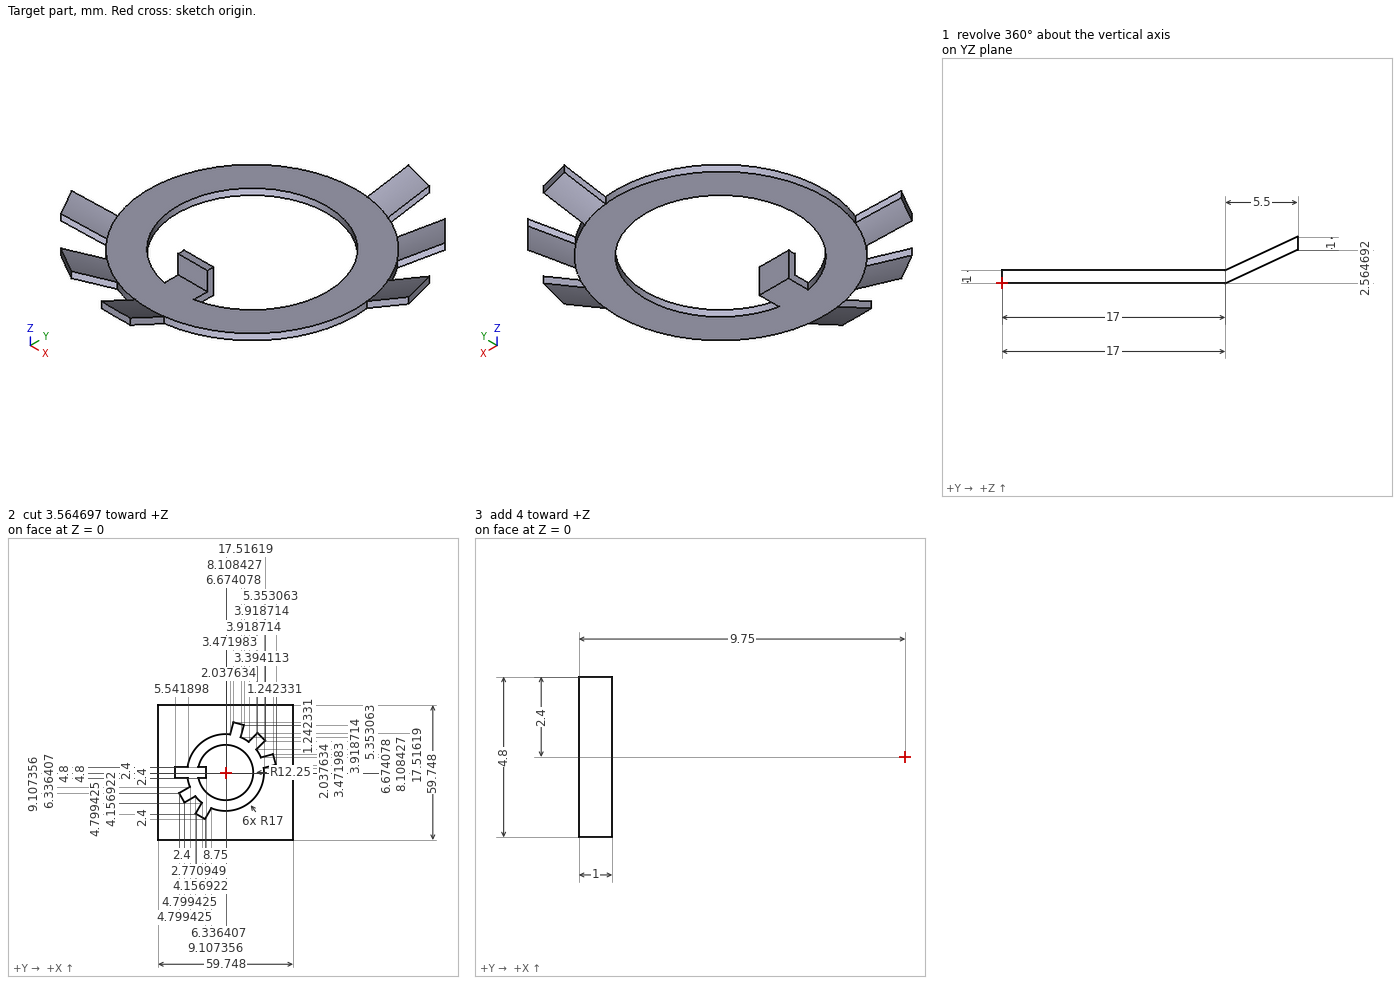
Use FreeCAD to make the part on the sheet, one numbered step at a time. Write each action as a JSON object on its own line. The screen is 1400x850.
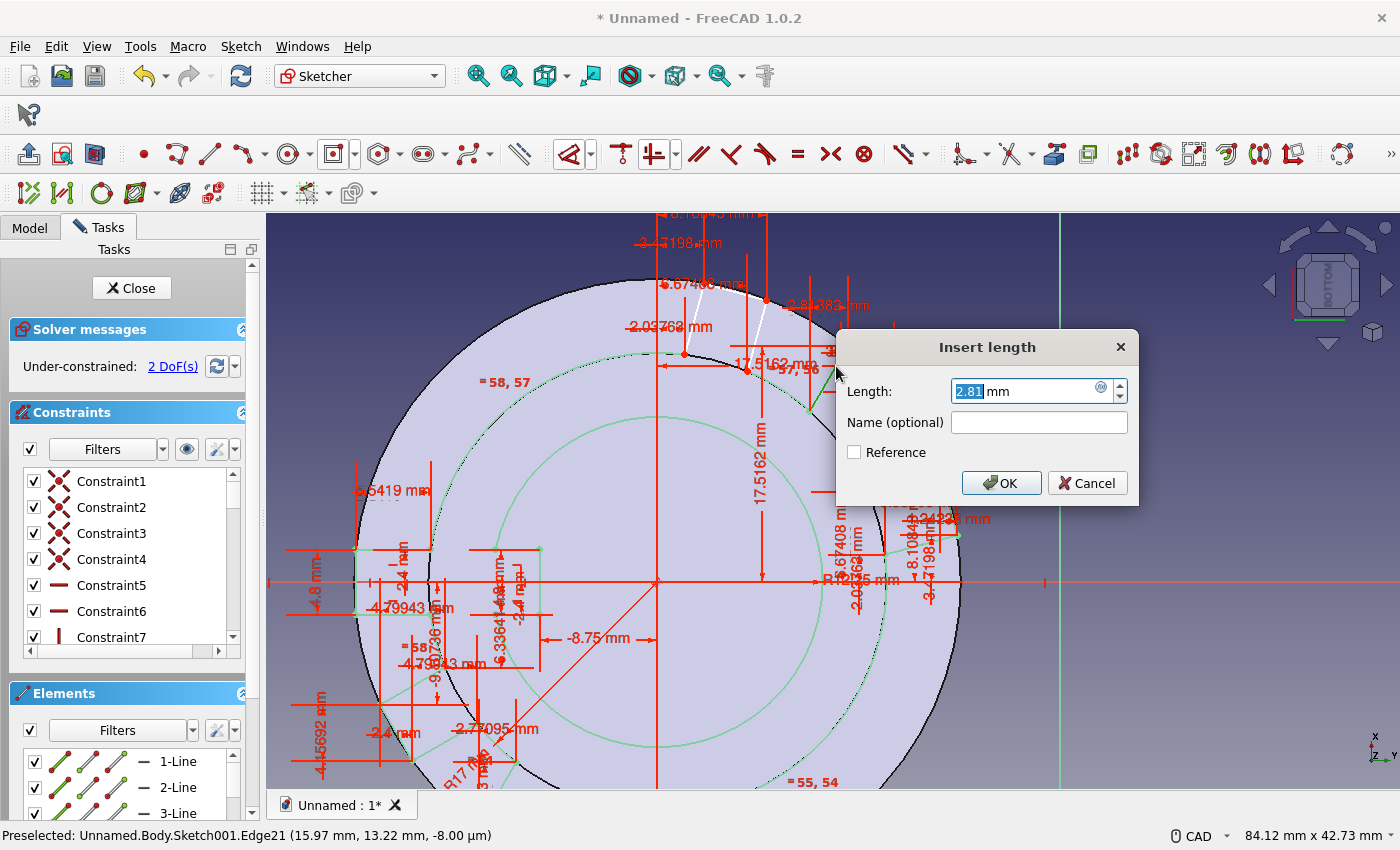
{"action": "type", "text": "3.918714"}
{"action": "key", "text": "Return"}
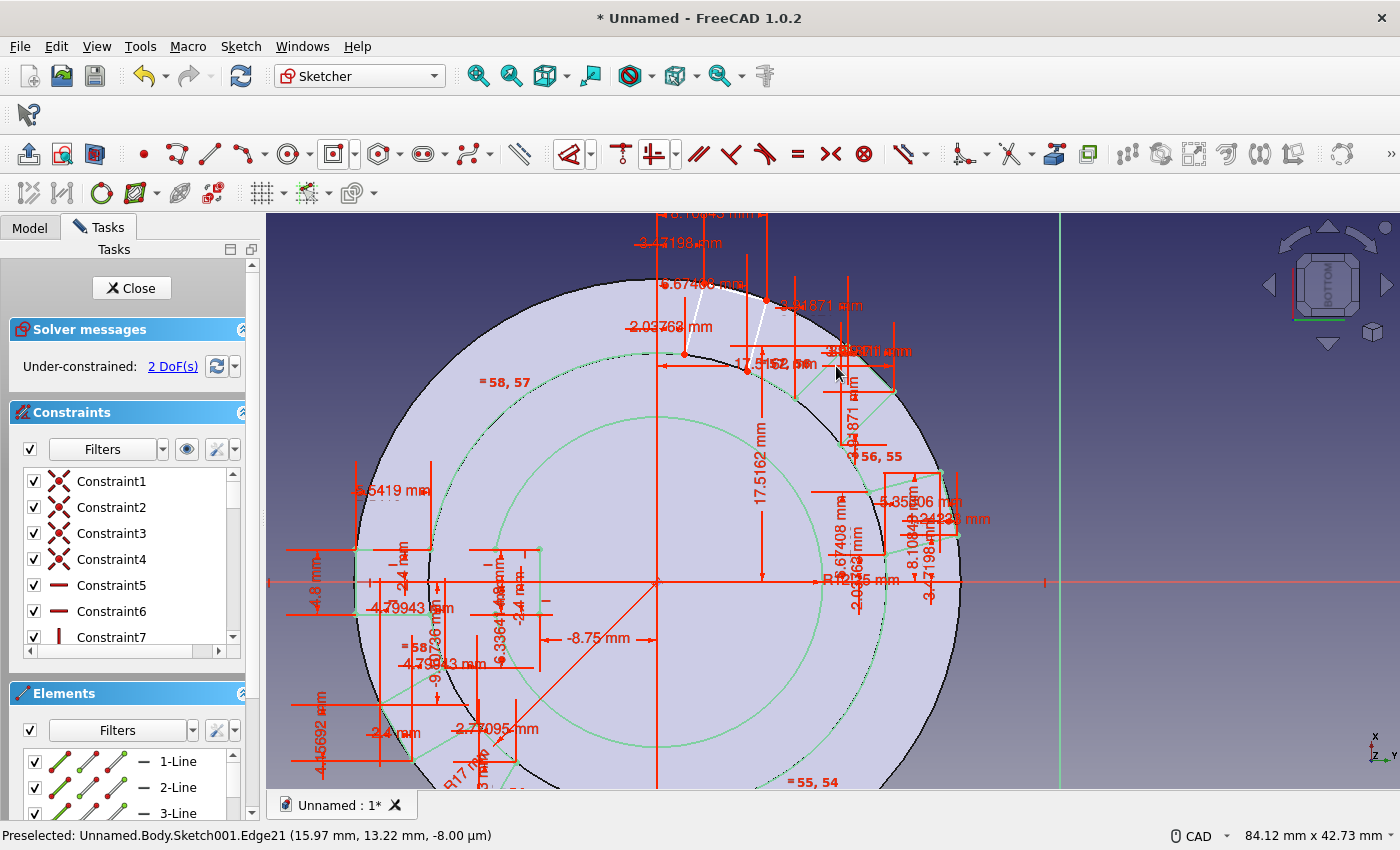
{"action": "left_click", "coordinate": [753, 350]}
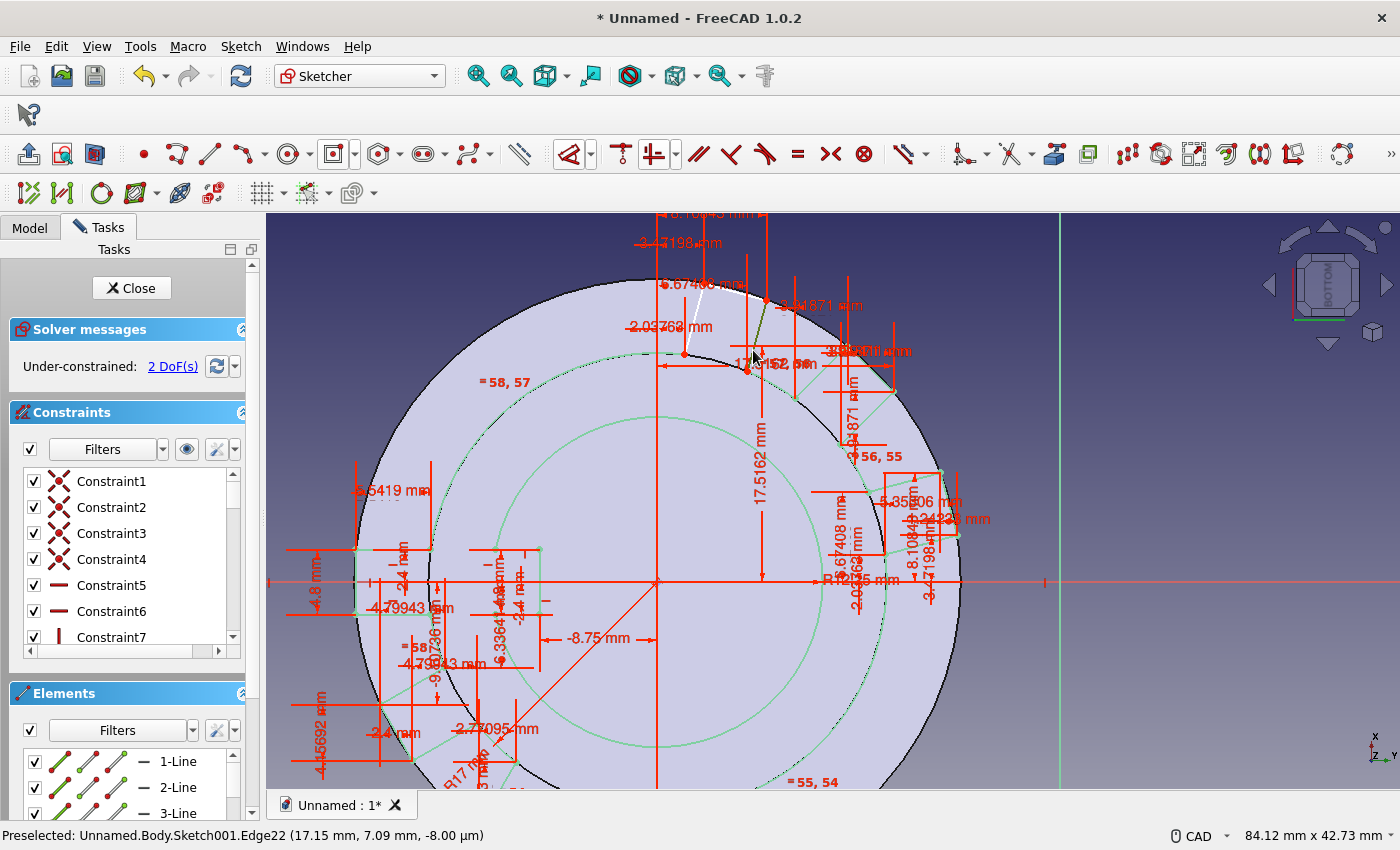
{"action": "key", "text": "i"}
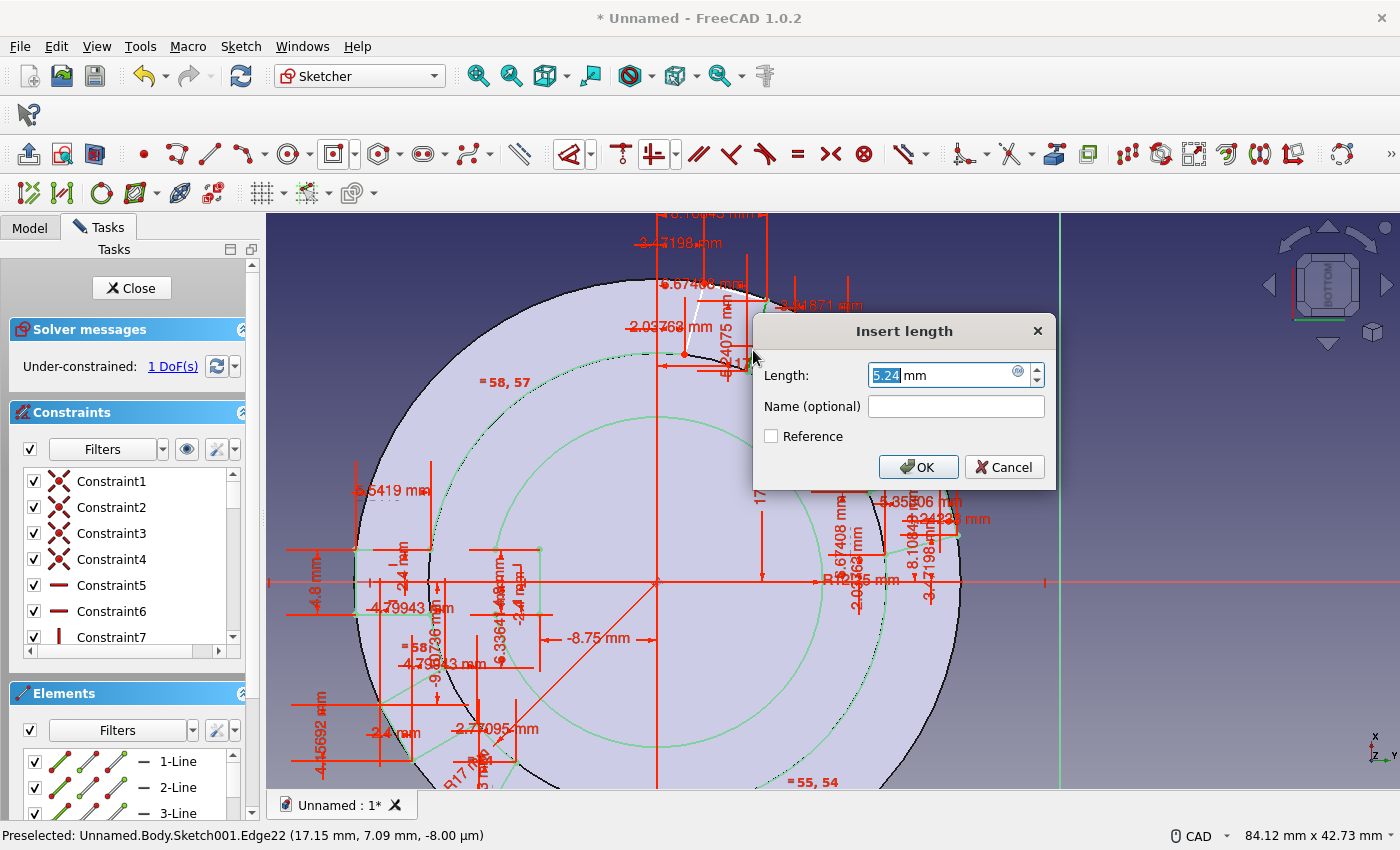
{"action": "type", "text": "5.353063"}
{"action": "key", "text": "Return"}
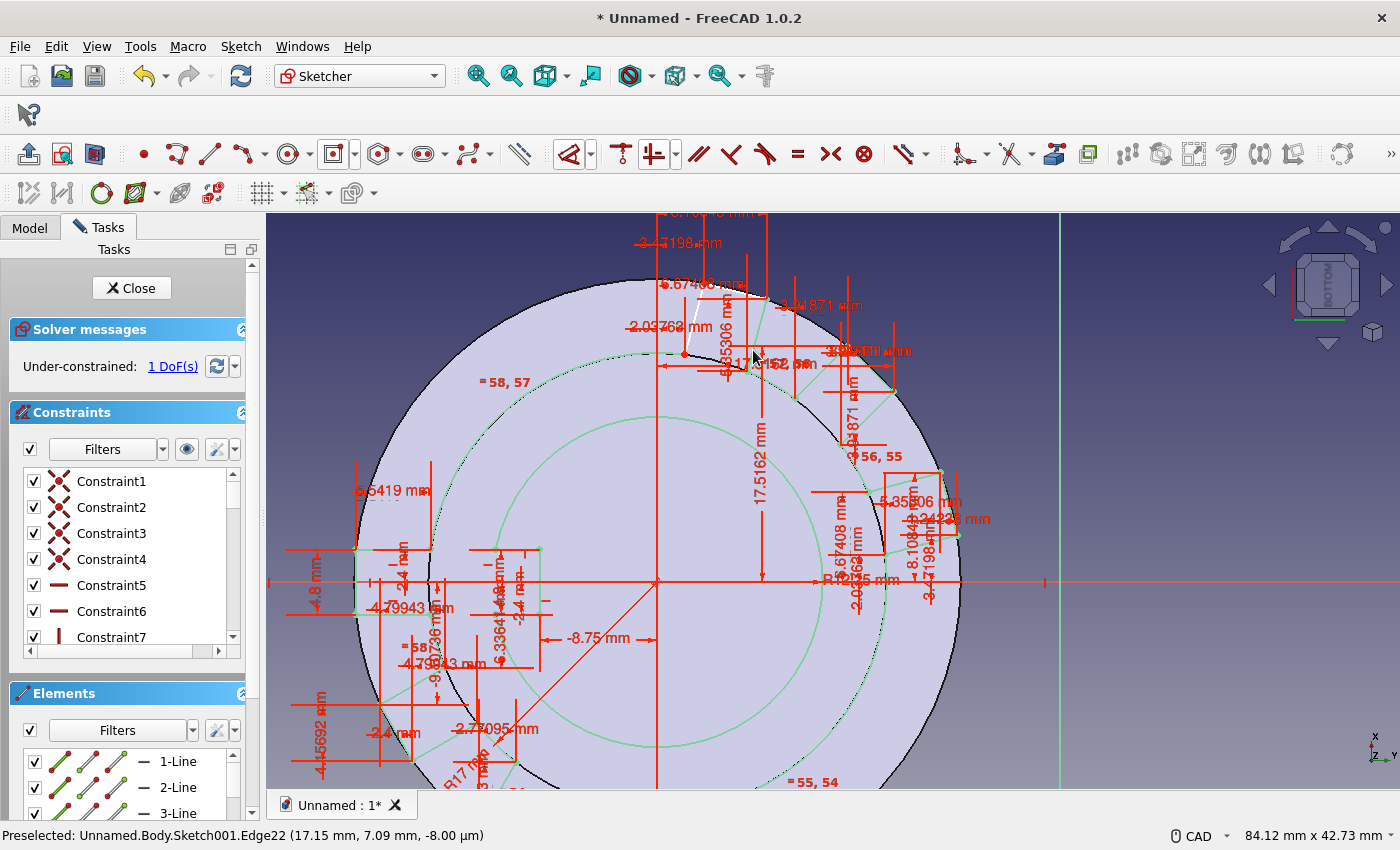
{"action": "scroll", "coordinate": [748, 295], "scroll_direction": "up", "scroll_amount": 5}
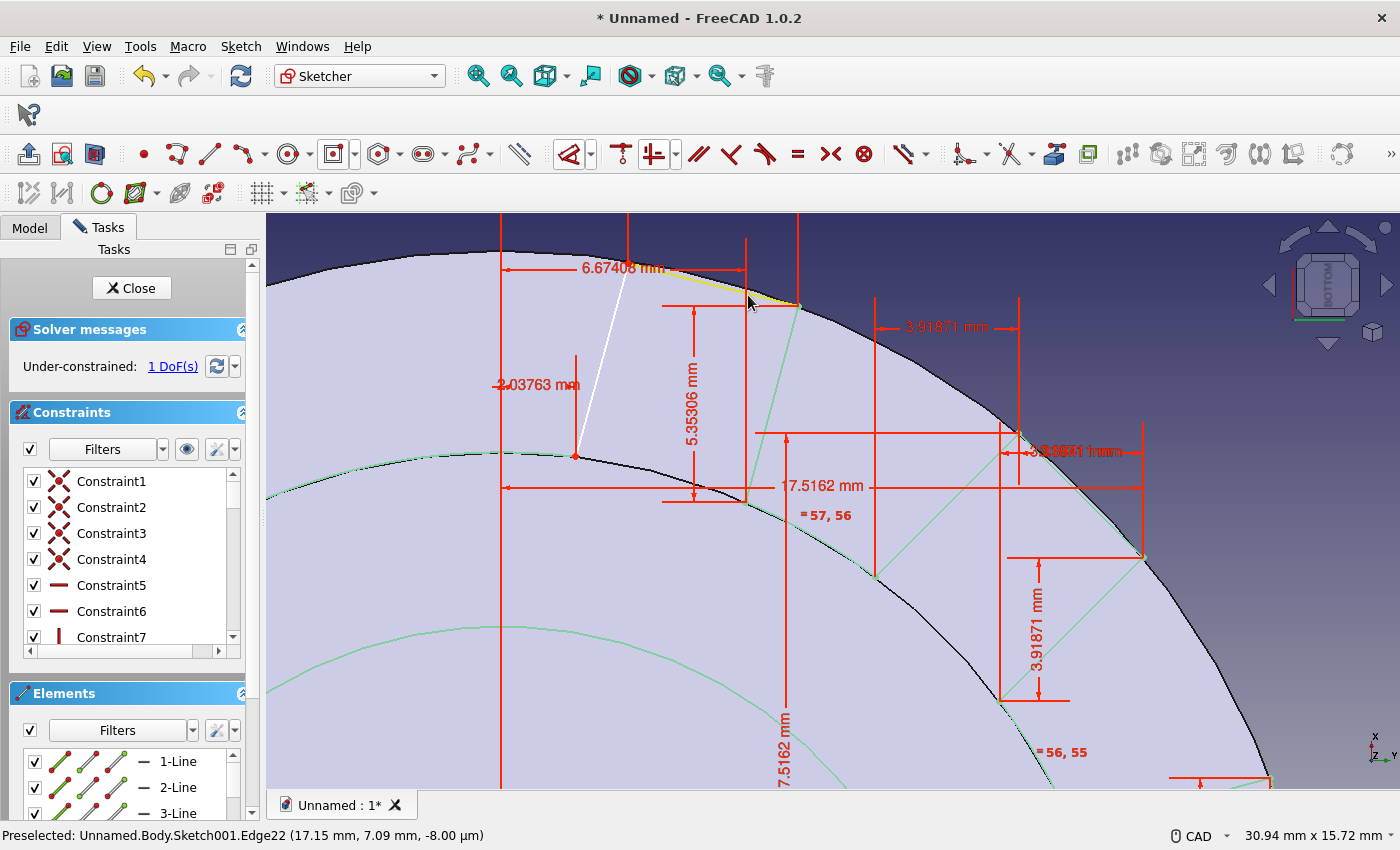
{"action": "left_click", "coordinate": [747, 293]}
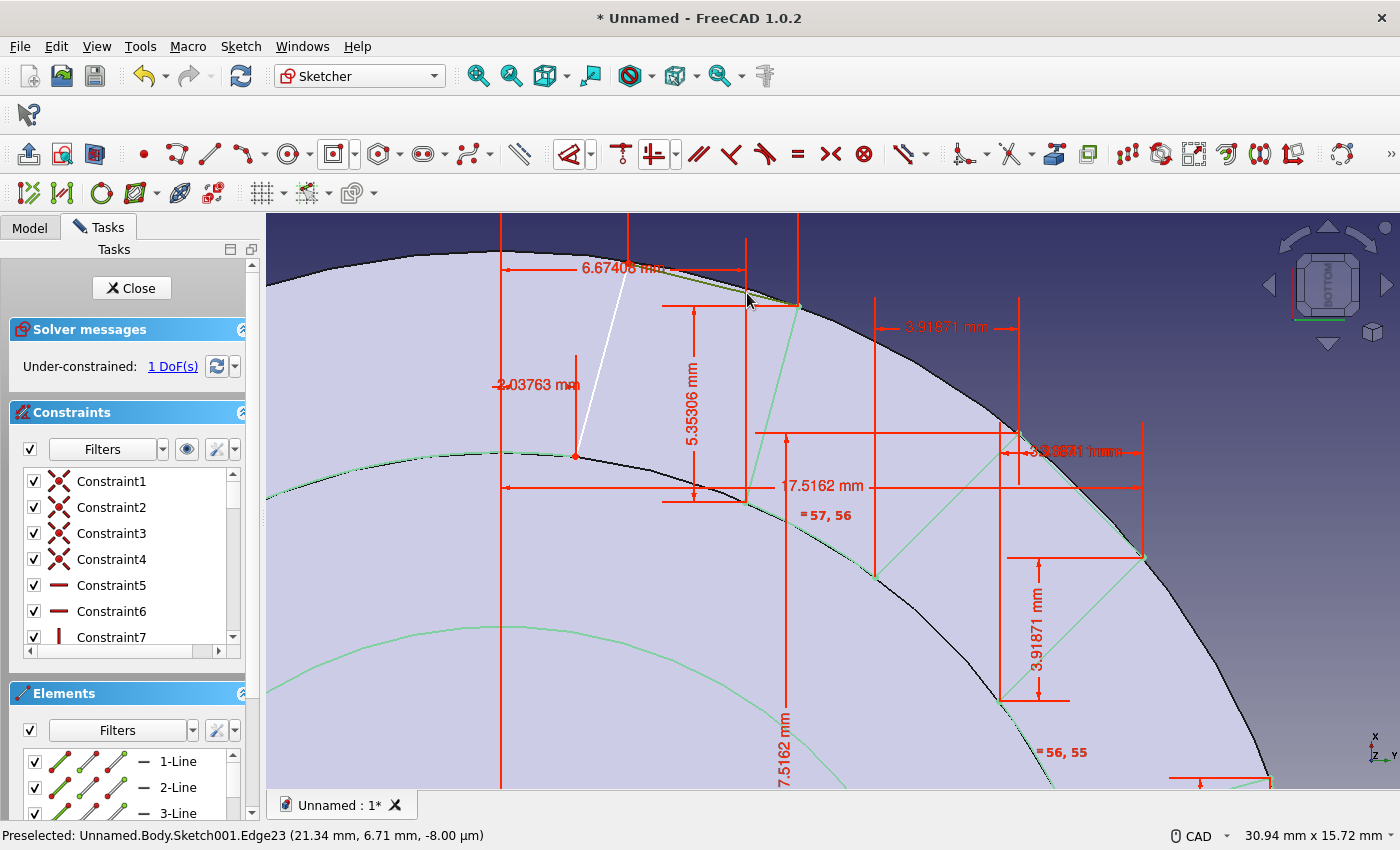
{"action": "left_click", "coordinate": [590, 154]}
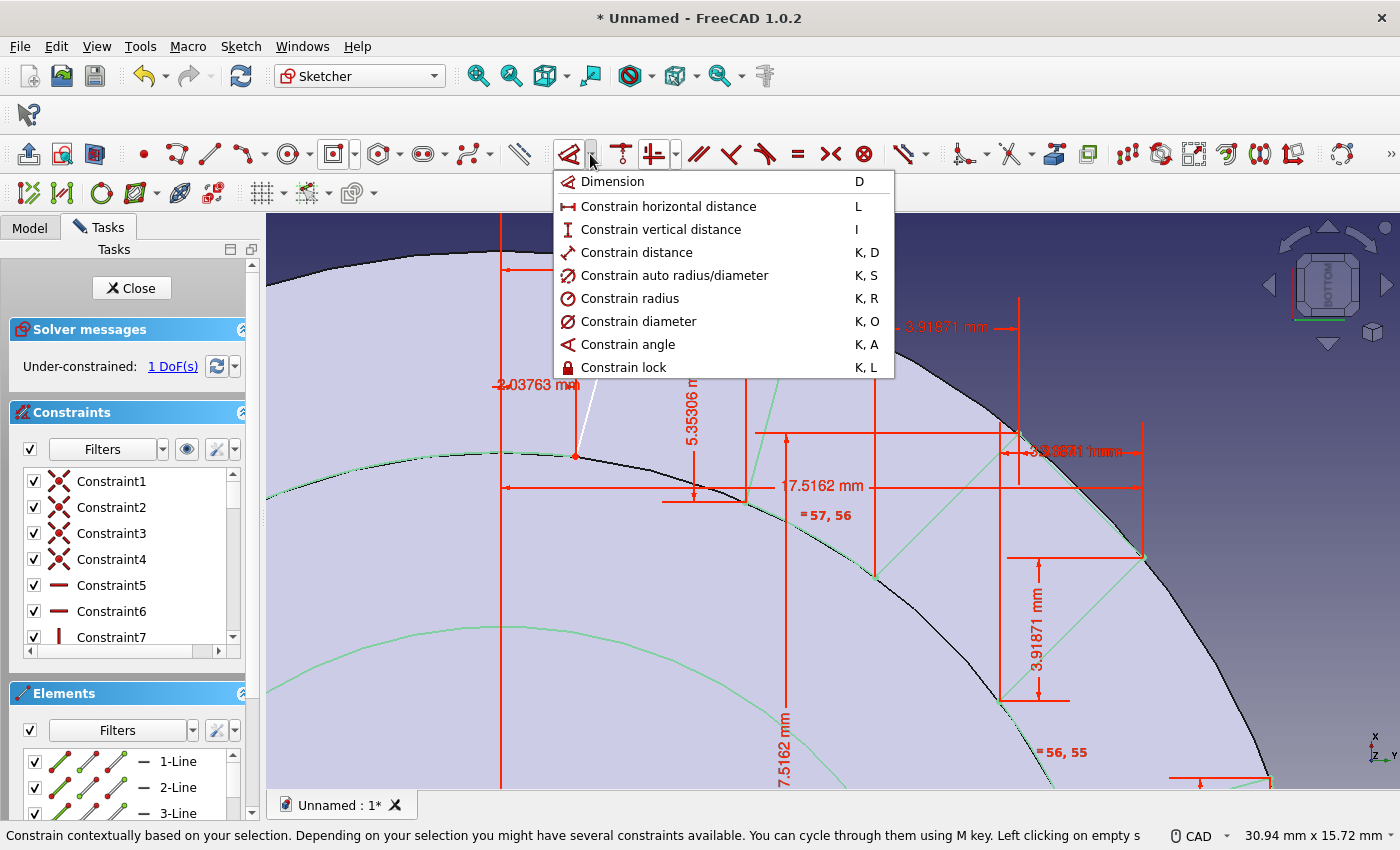
{"action": "left_click", "coordinate": [724, 230]}